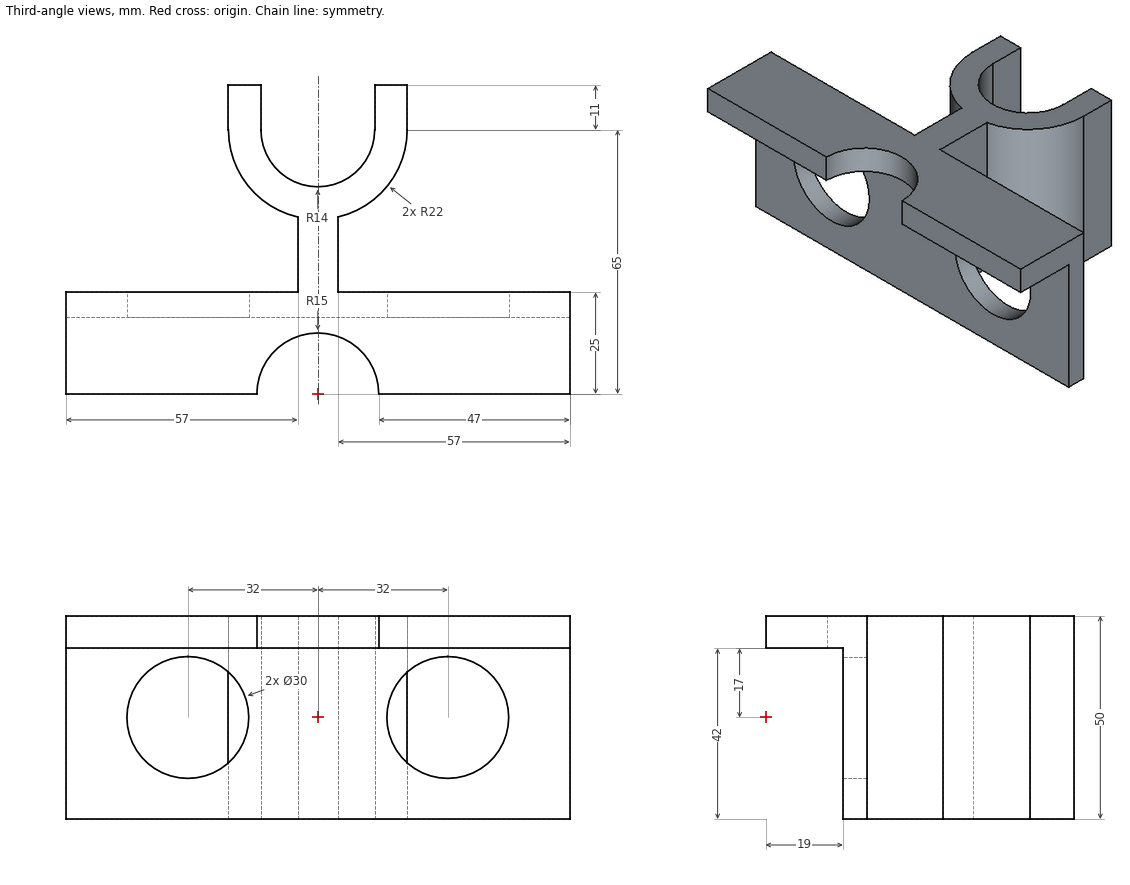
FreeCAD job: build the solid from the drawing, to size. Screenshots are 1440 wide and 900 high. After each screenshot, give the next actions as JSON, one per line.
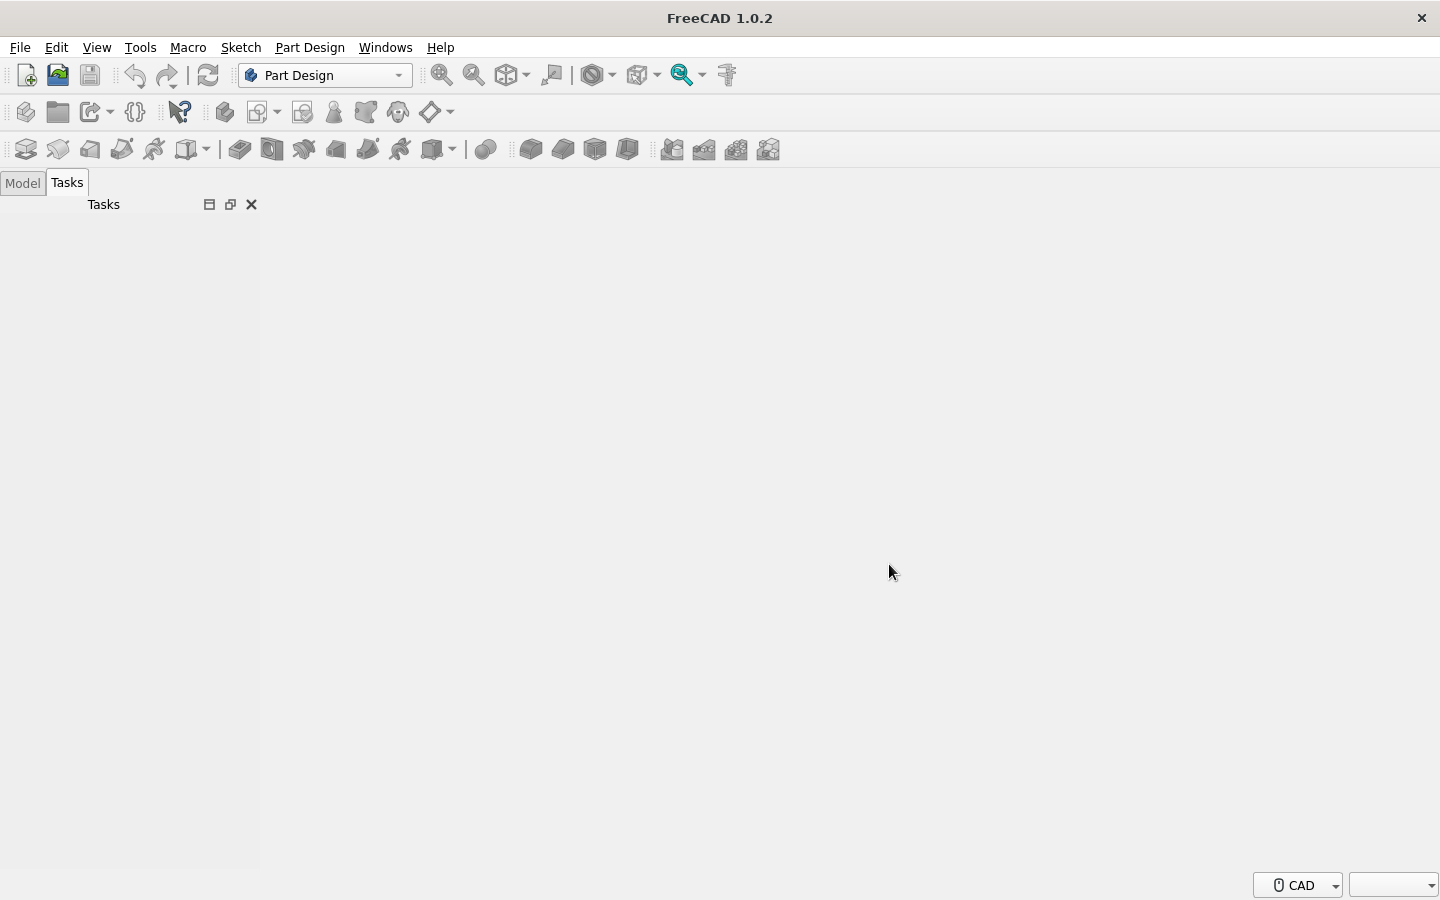
{"action": "left_click", "coordinate": [26, 76]}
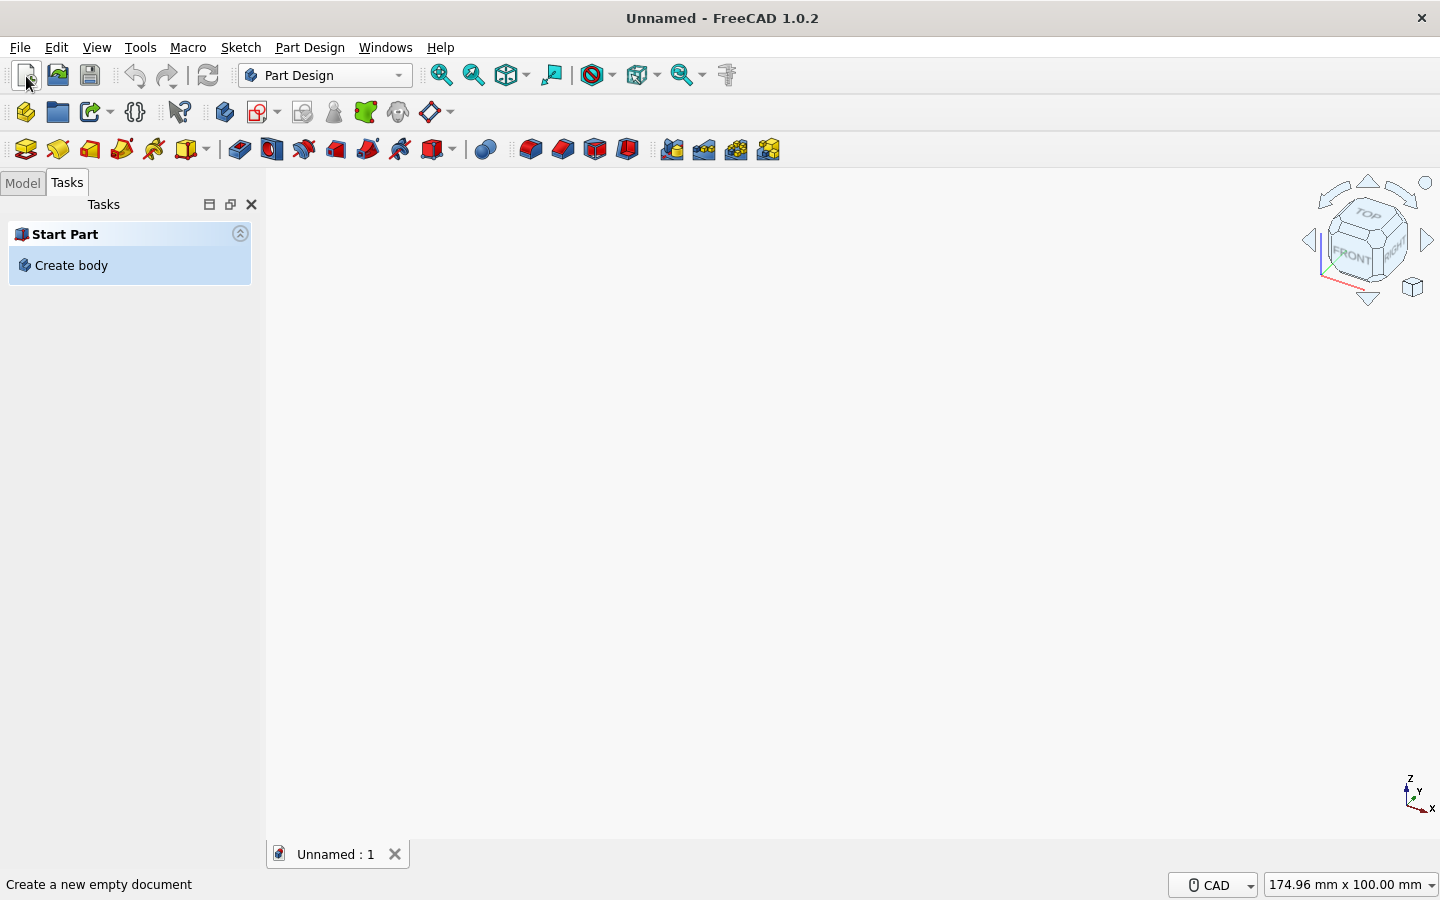
{"action": "left_click", "coordinate": [258, 112]}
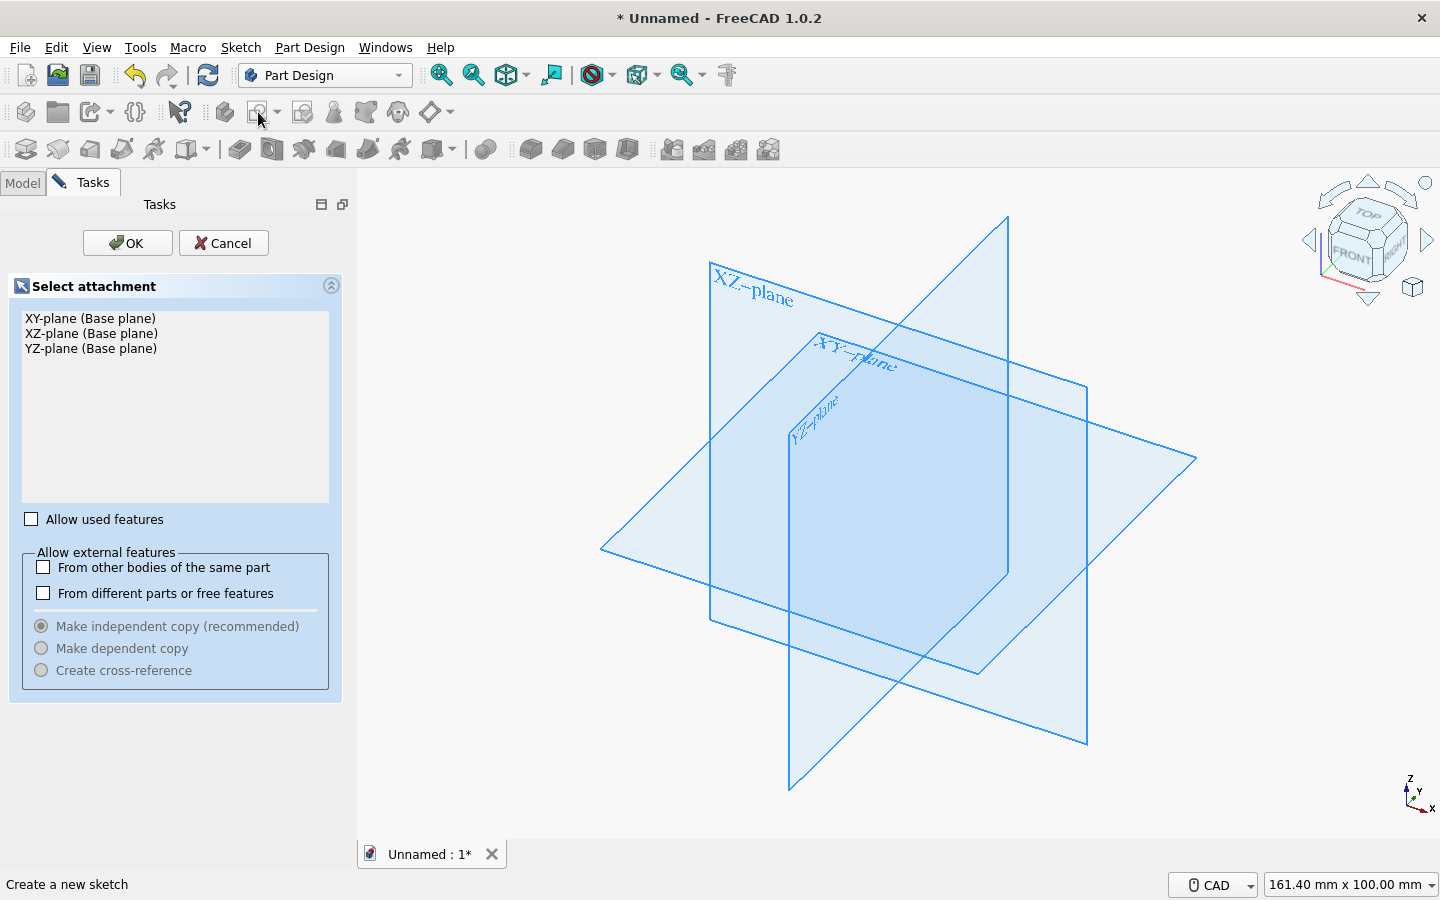
{"action": "left_click", "coordinate": [82, 318]}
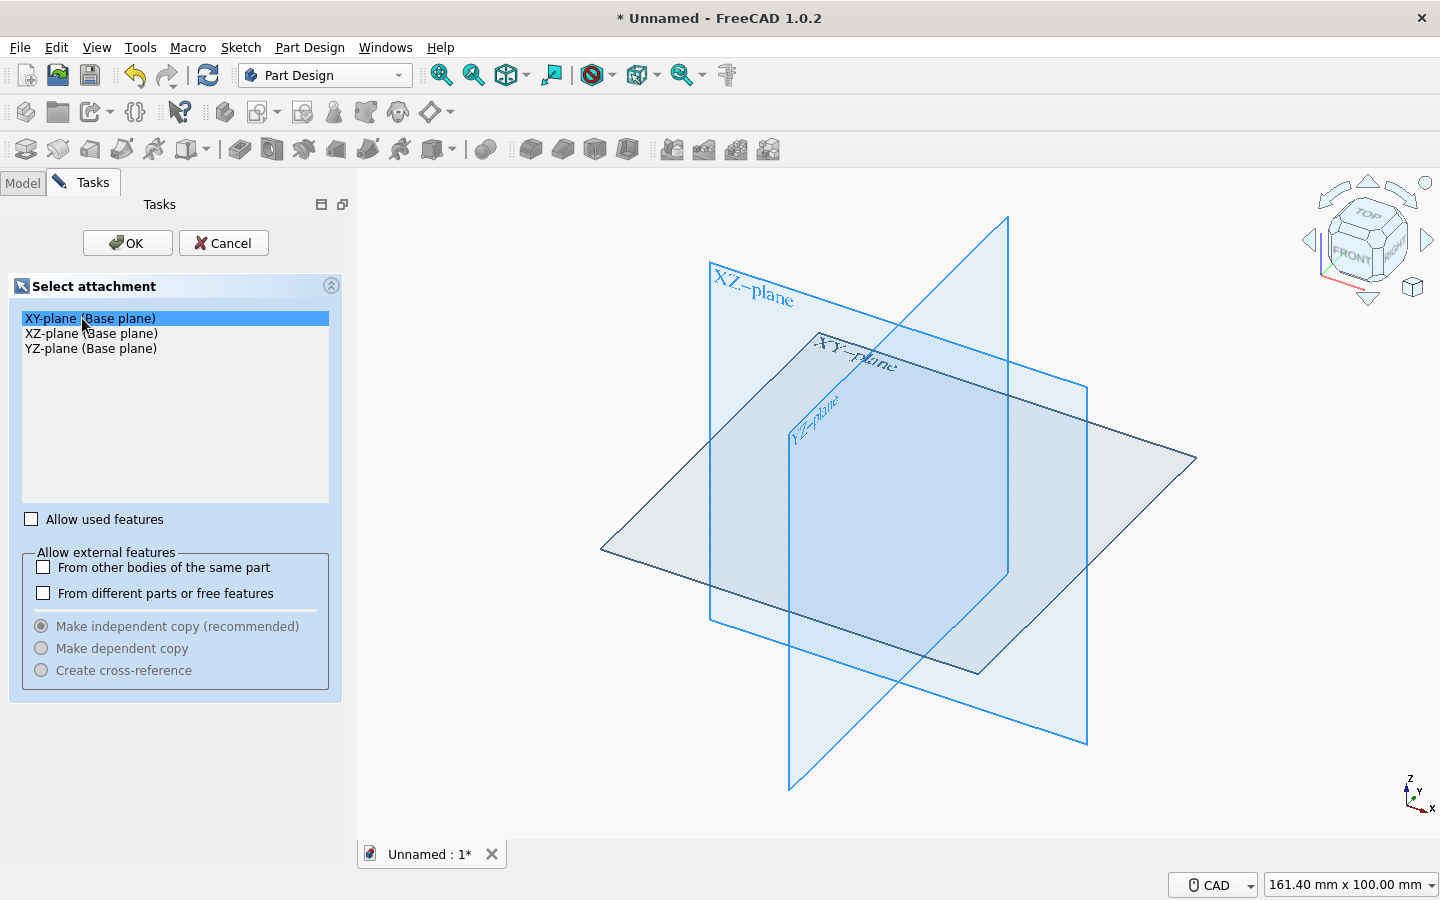
{"action": "left_click", "coordinate": [128, 243]}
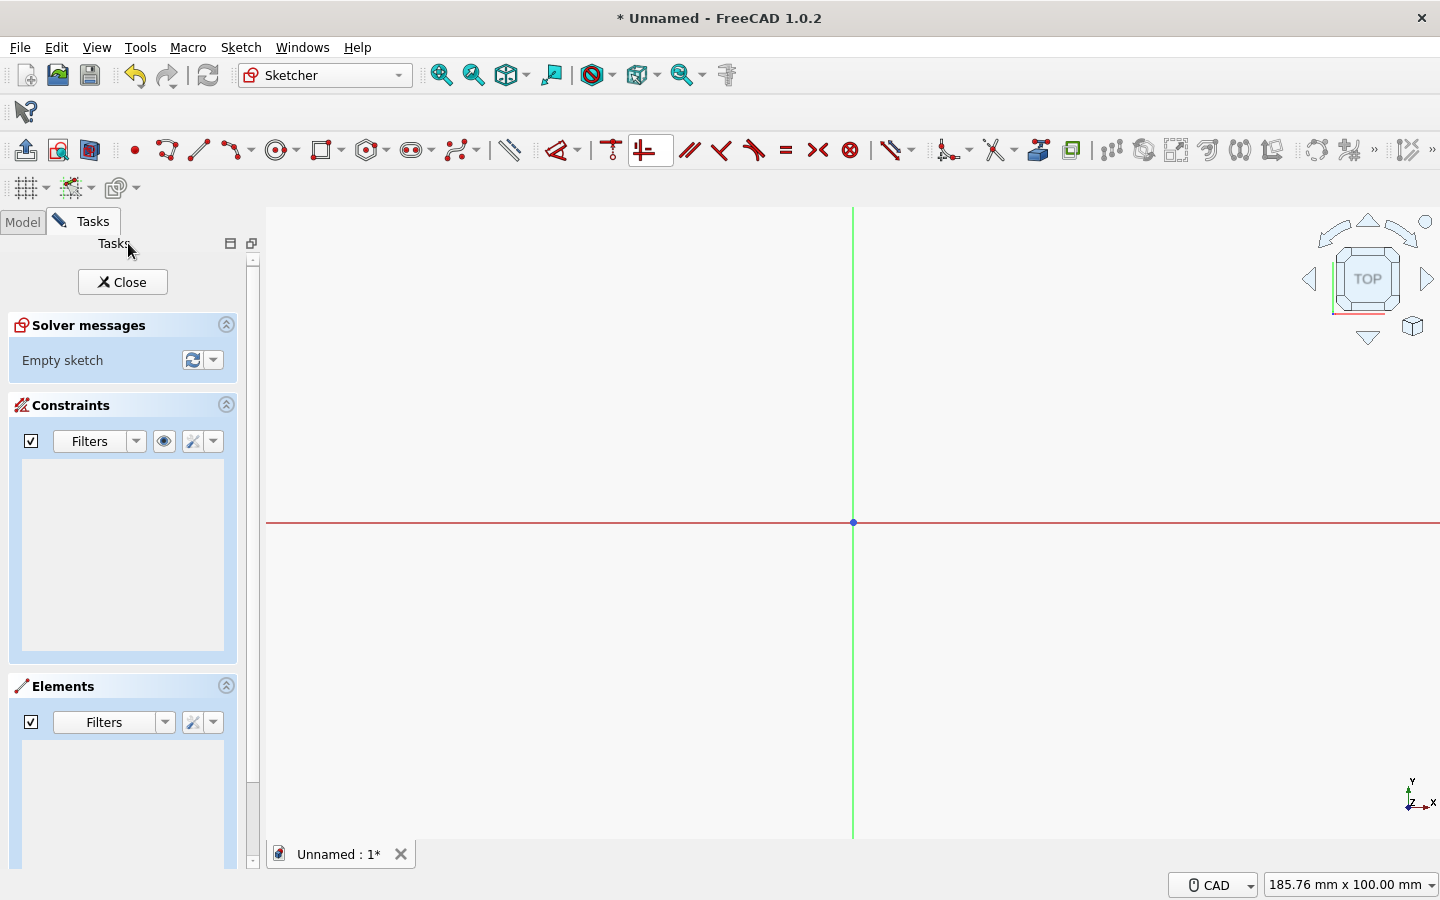
{"action": "scroll", "coordinate": [645, 811], "scroll_direction": "down", "scroll_amount": 2}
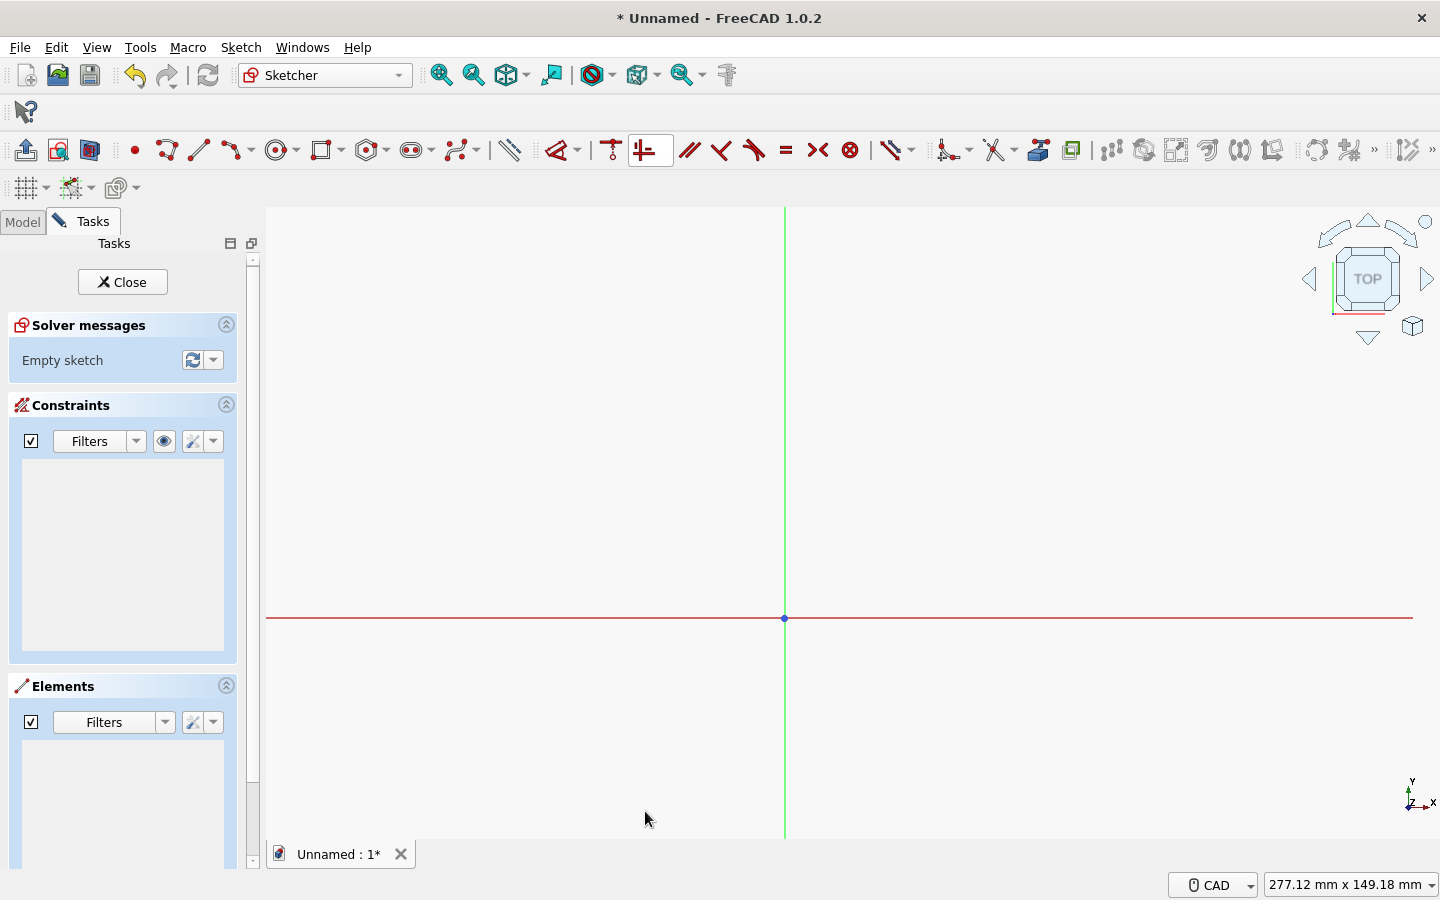
{"action": "left_click", "coordinate": [168, 150]}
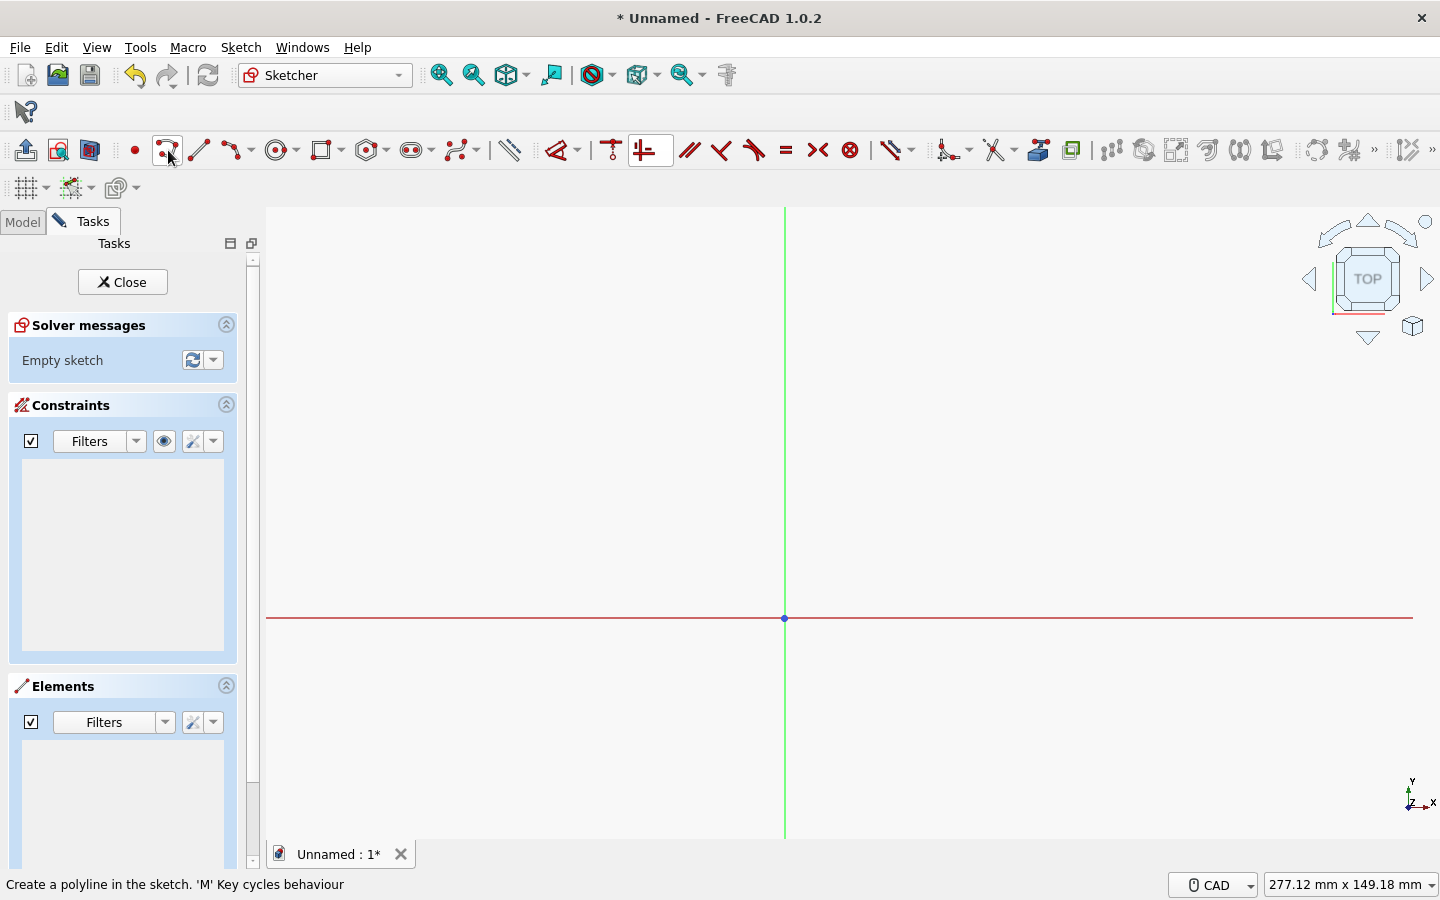
{"action": "left_click", "coordinate": [848, 618]}
{"action": "left_click", "coordinate": [1047, 609]}
{"action": "left_click", "coordinate": [1047, 512]}
{"action": "left_click", "coordinate": [806, 512]}
{"action": "left_click", "coordinate": [806, 434]}
{"action": "right_click", "coordinate": [806, 434]}